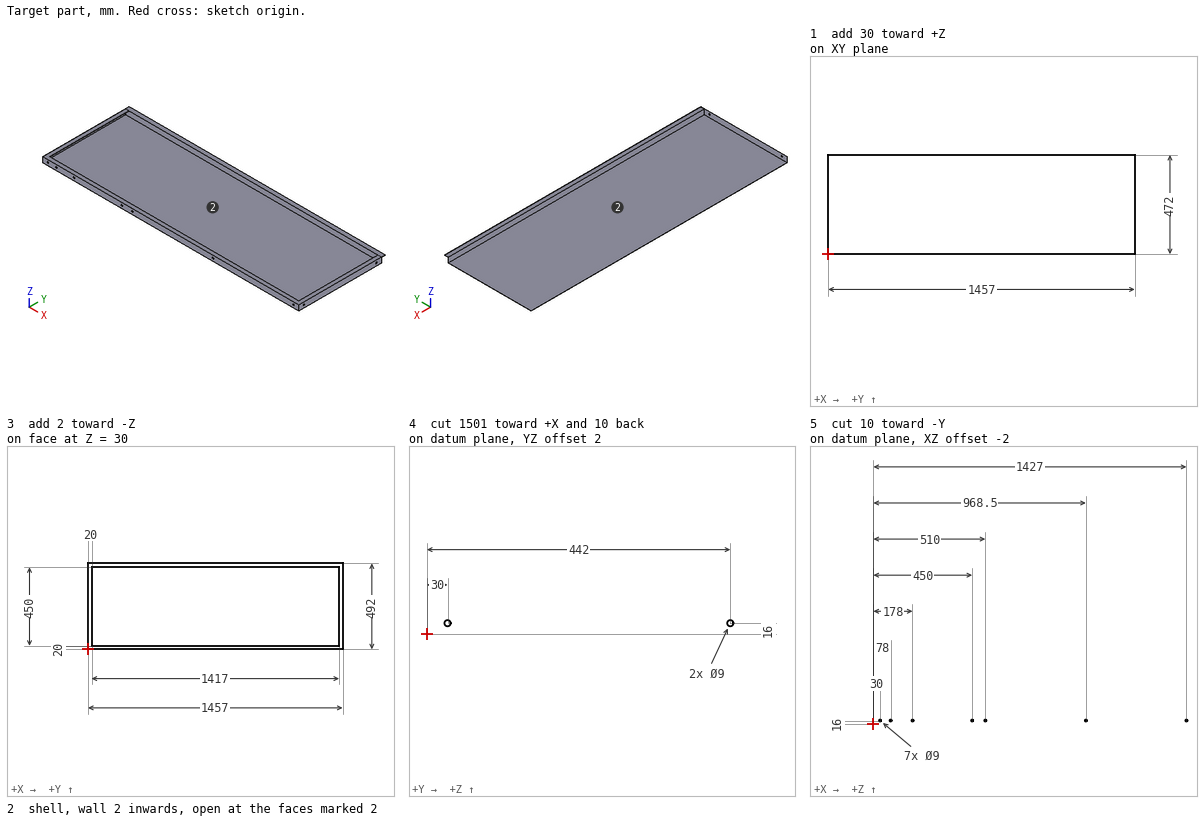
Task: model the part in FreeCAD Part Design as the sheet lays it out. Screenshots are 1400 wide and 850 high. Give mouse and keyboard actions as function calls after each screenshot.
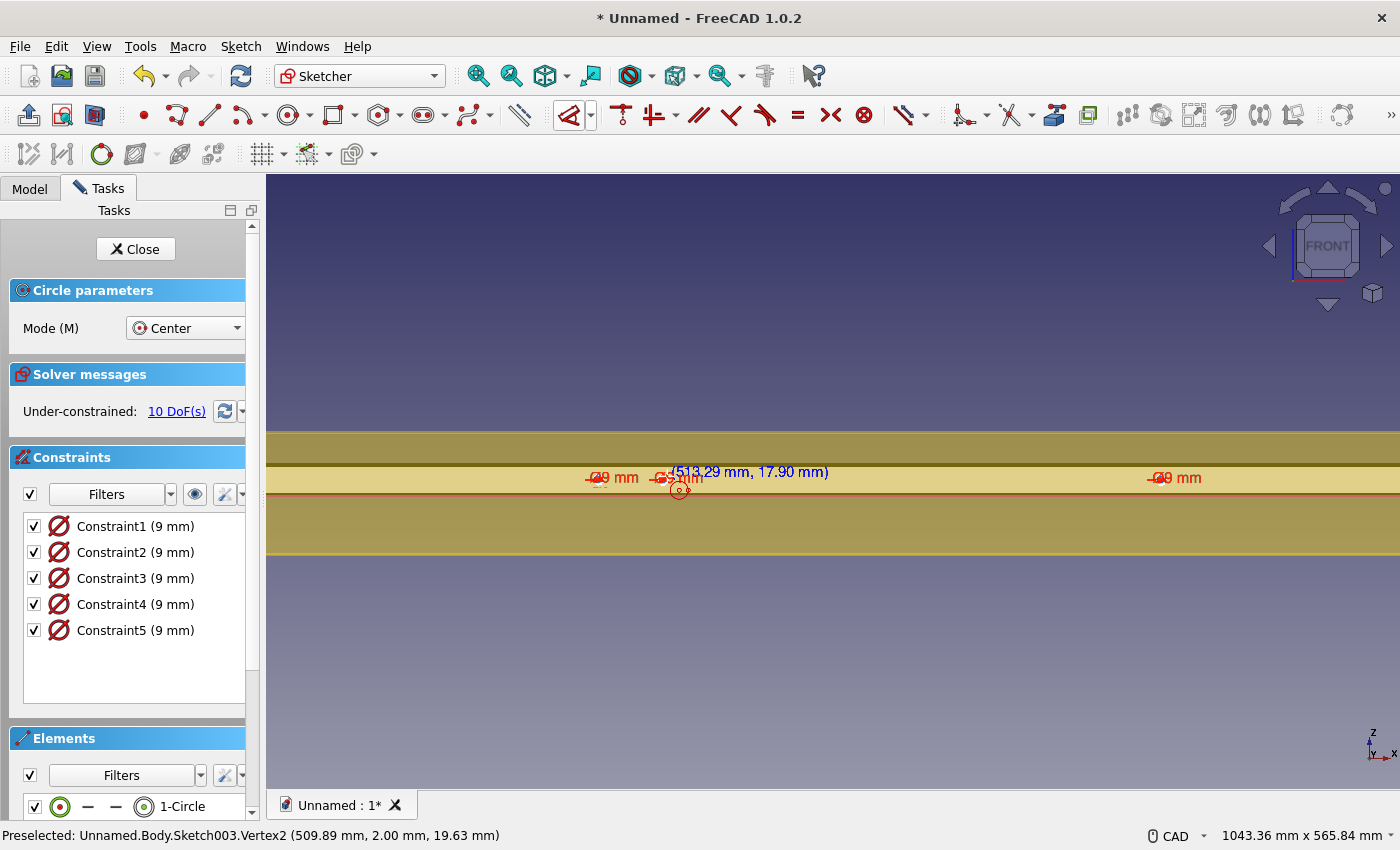
scroll(665, 478, down, 4)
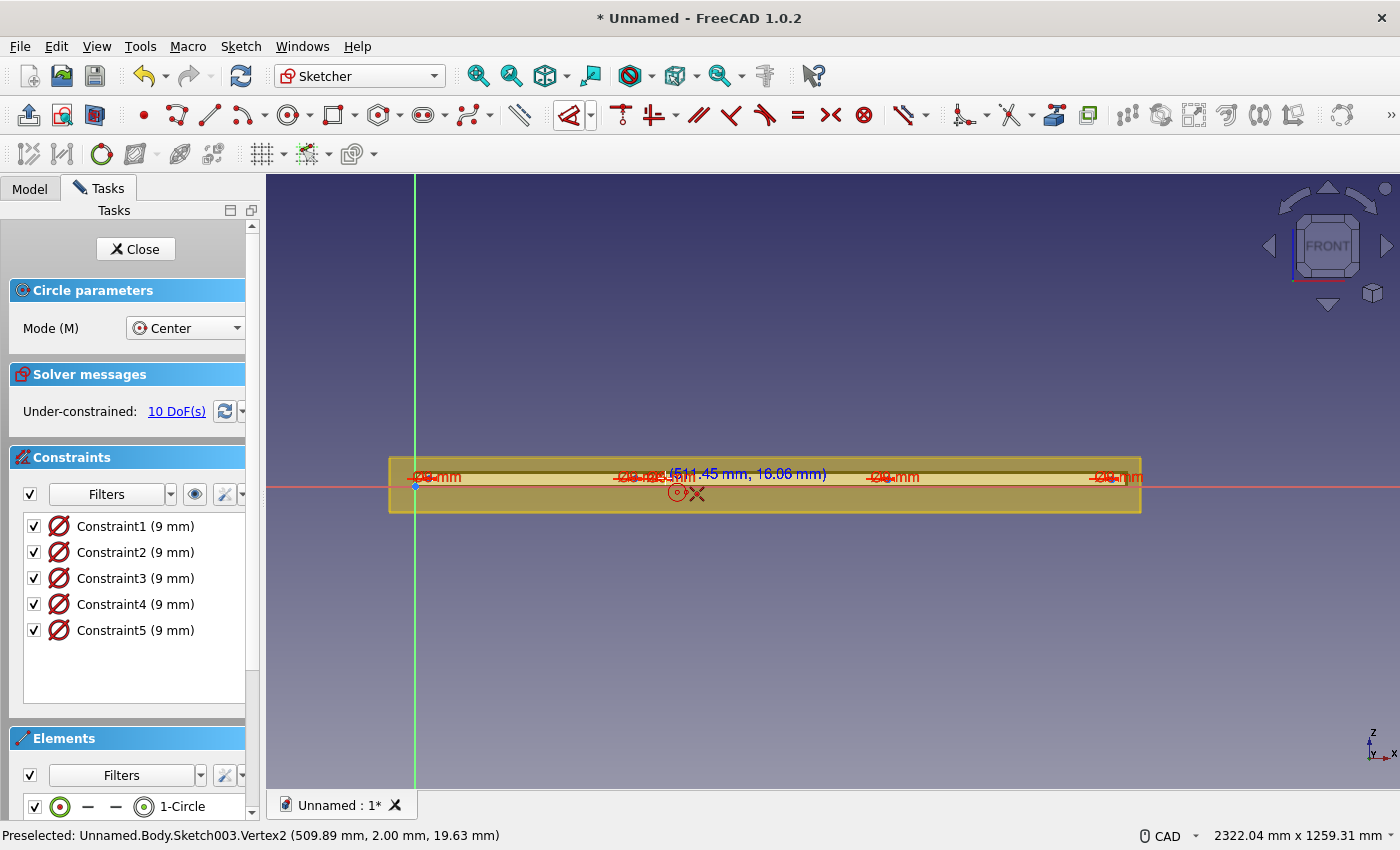
scroll(454, 479, up, 12)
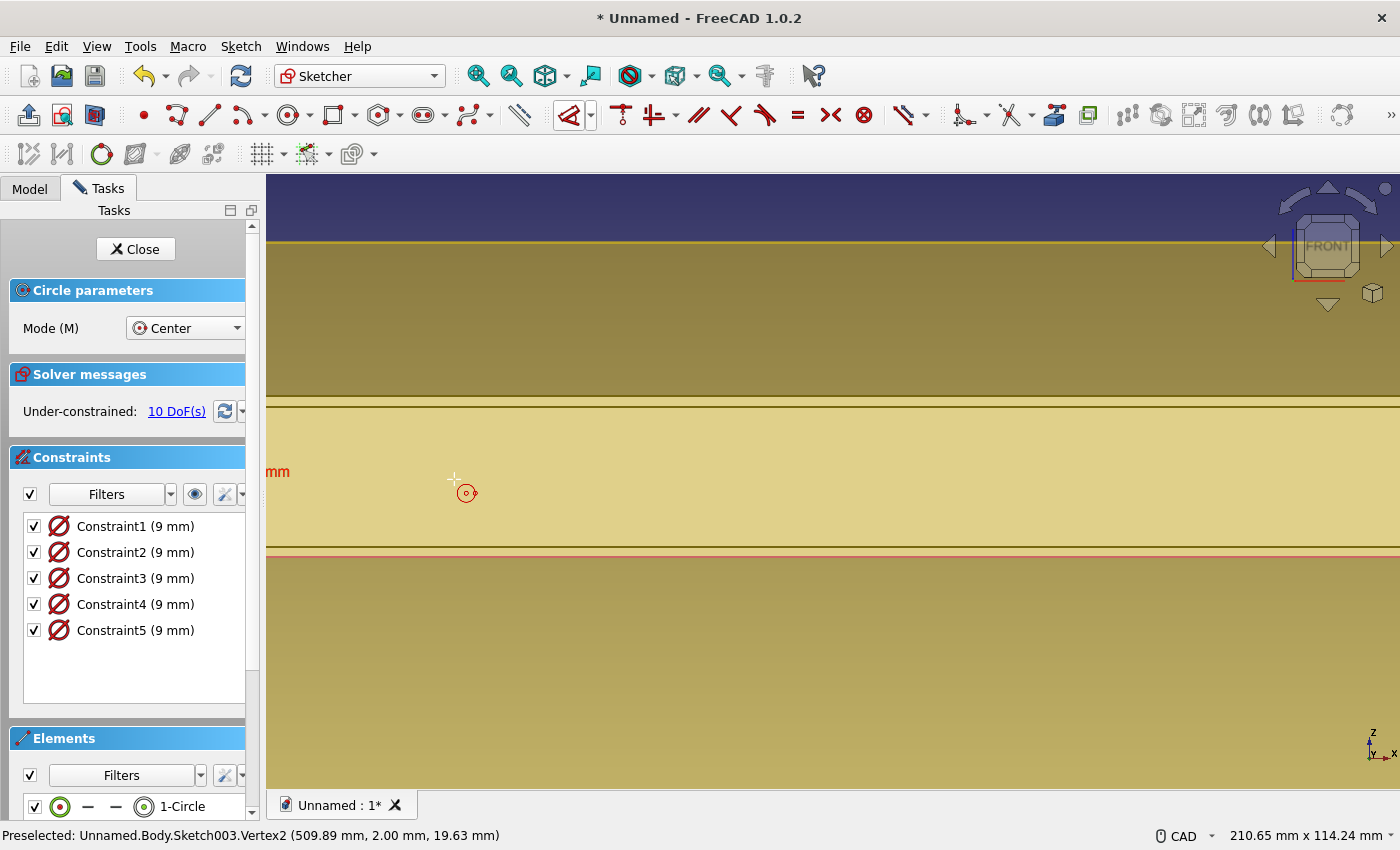
scroll(454, 479, down, 12)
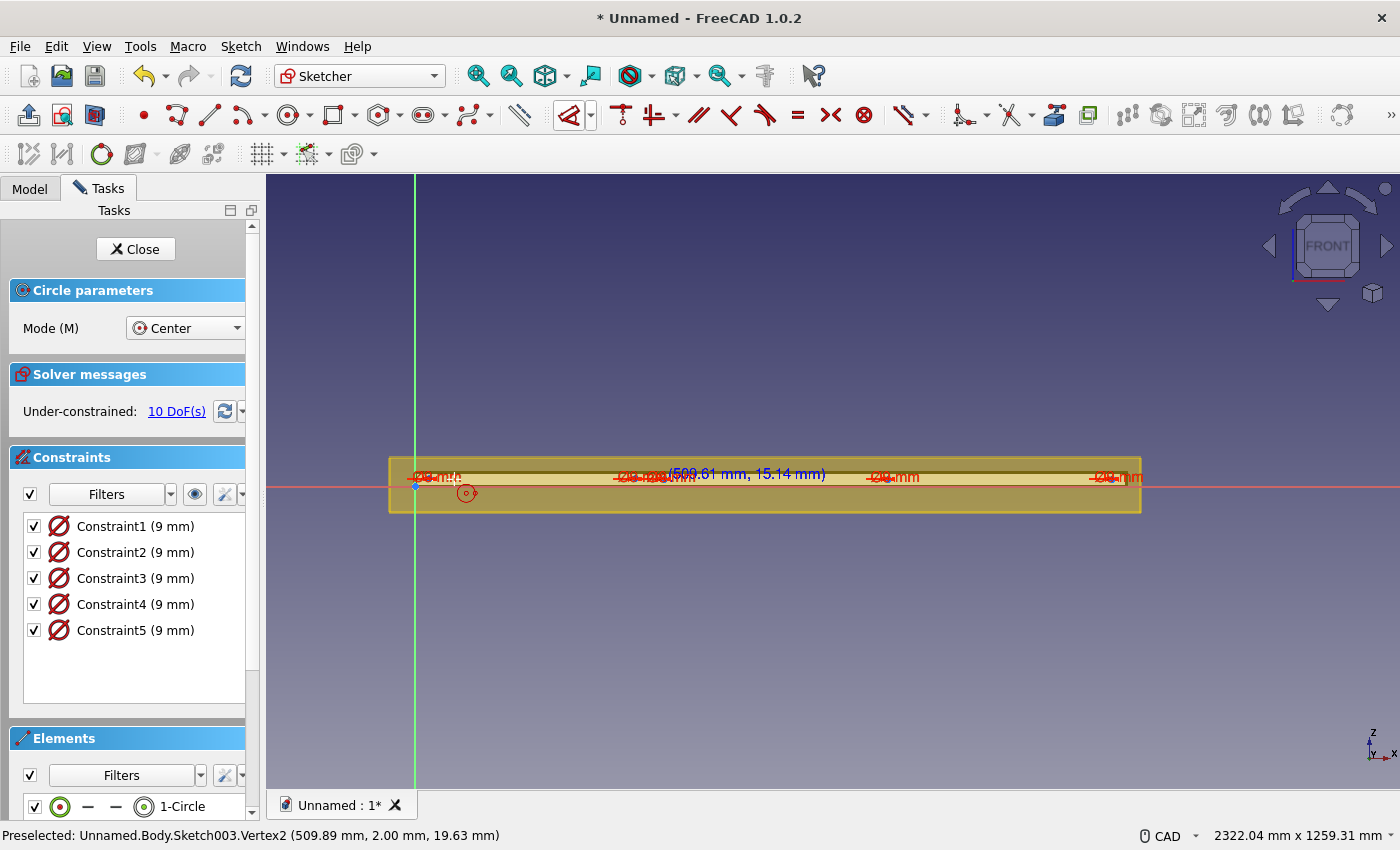
scroll(454, 479, up, 4)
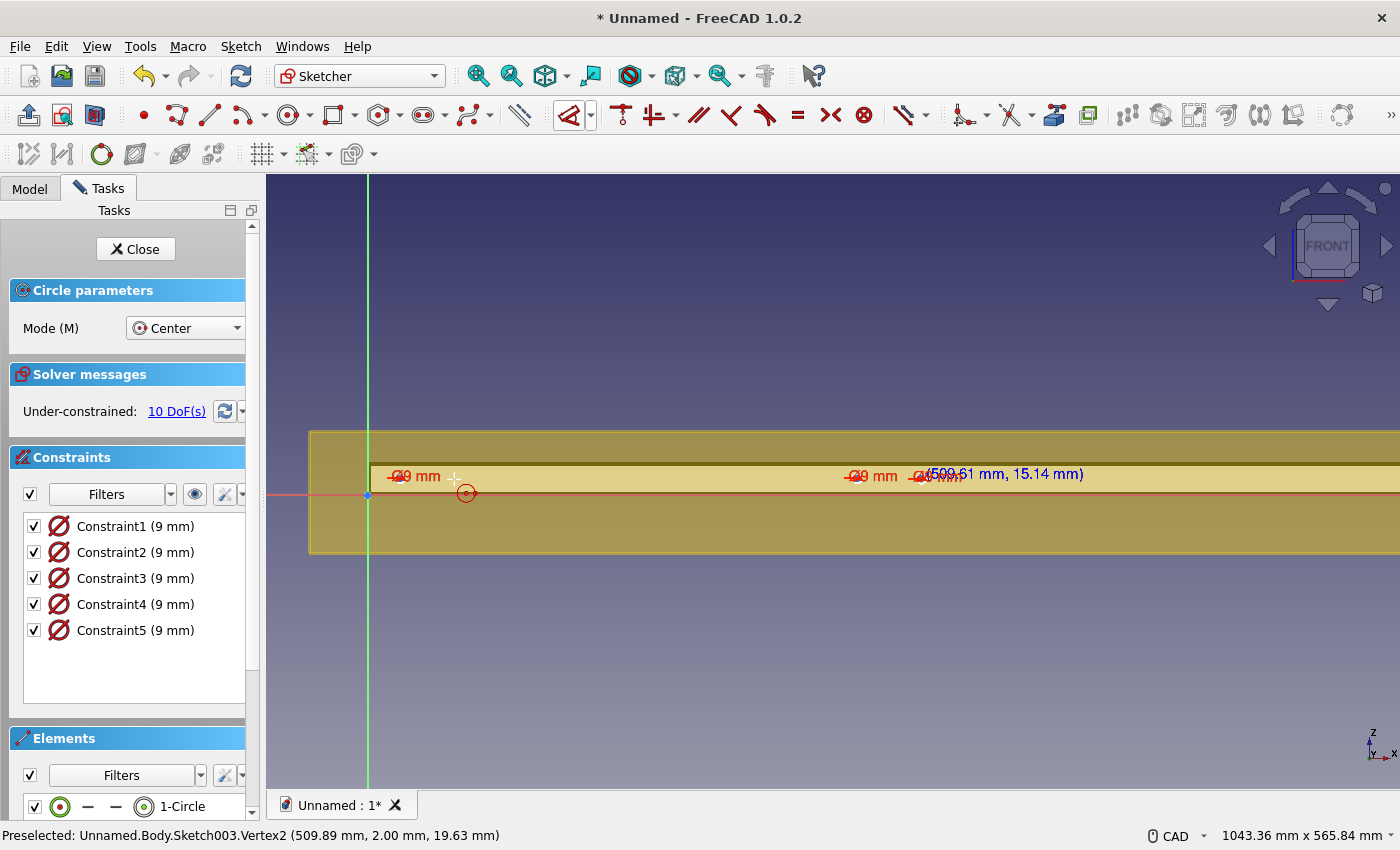
click(453, 478)
move(456, 474)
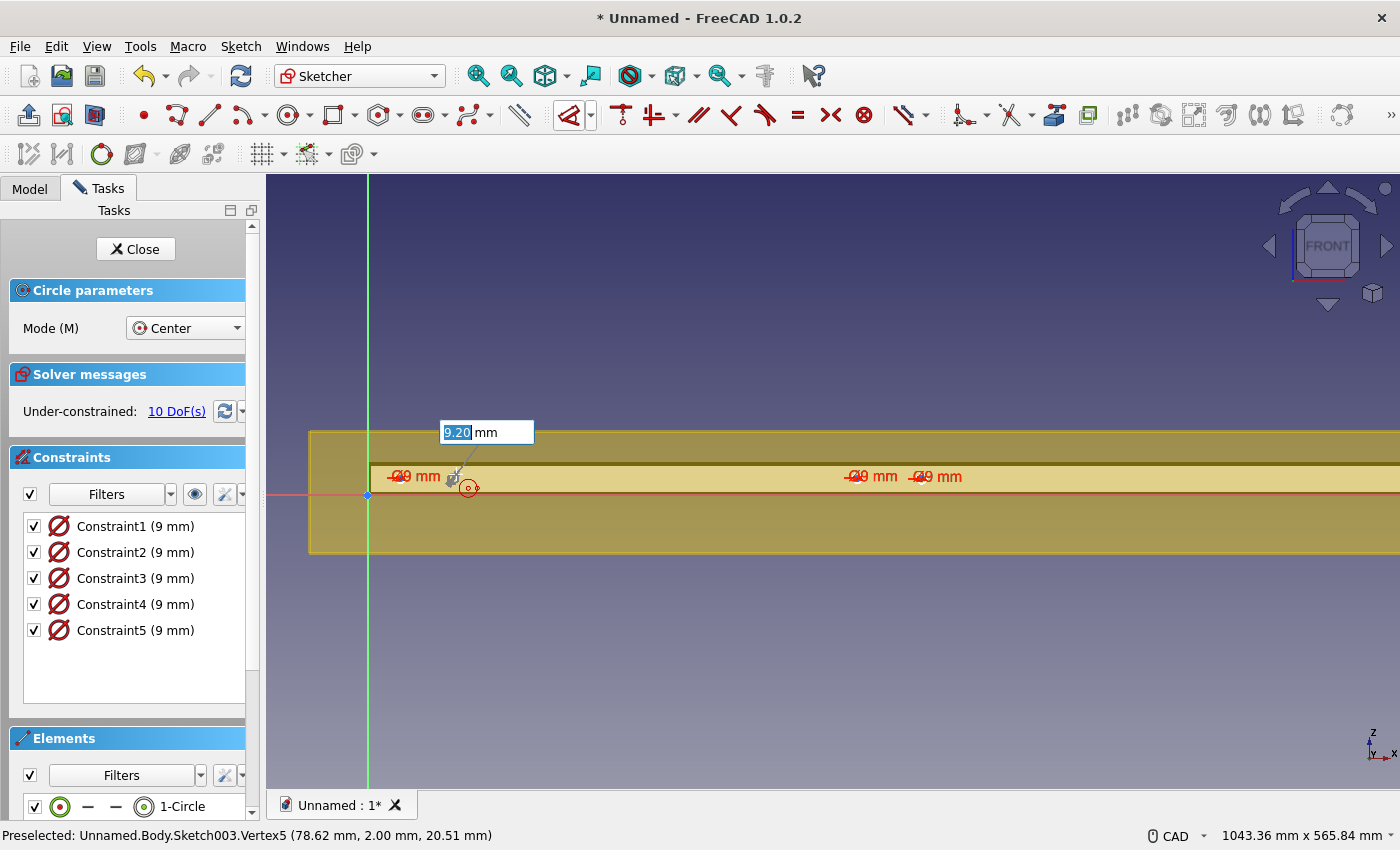
text(9)
key(Return)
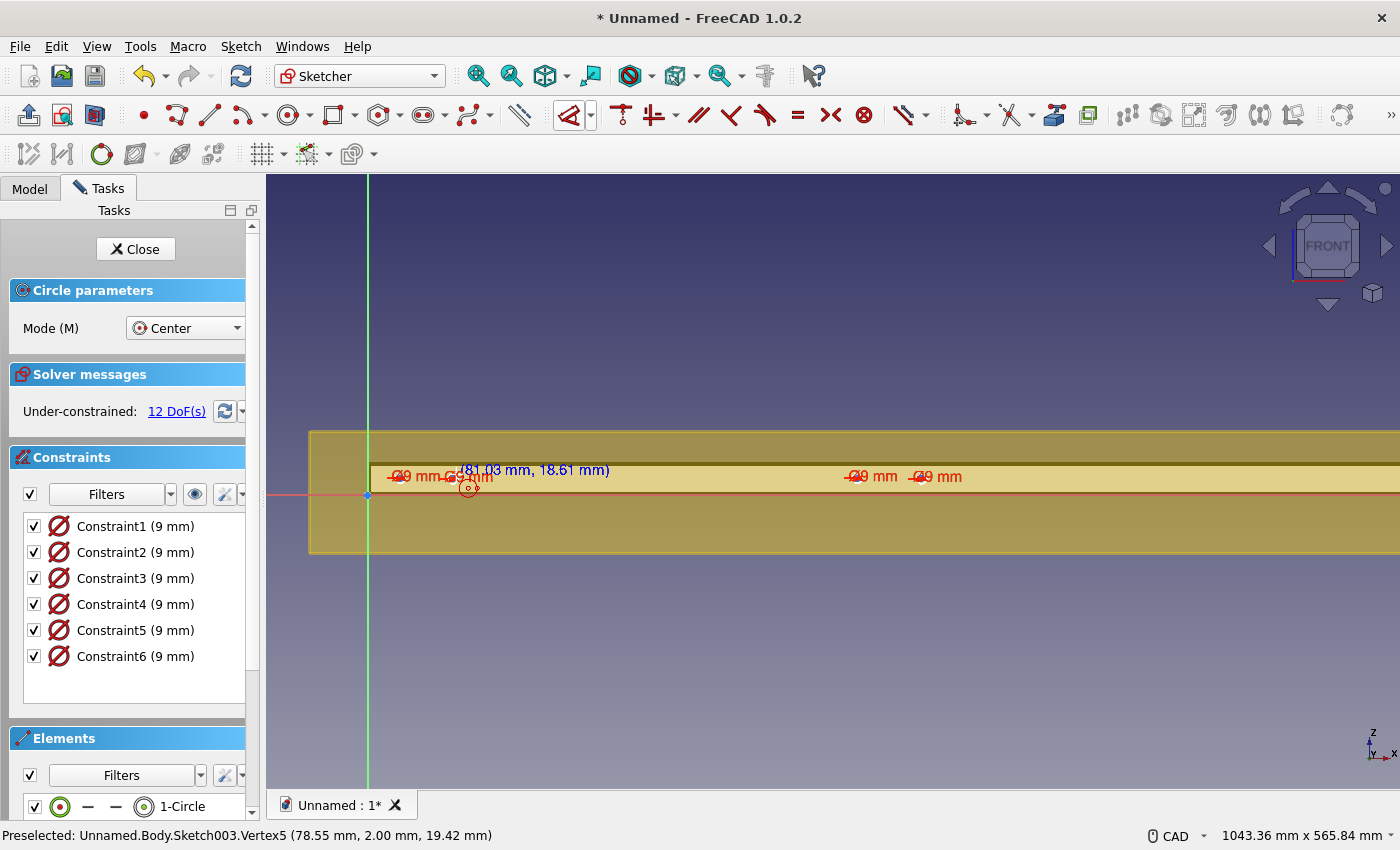
scroll(561, 478, up, 8)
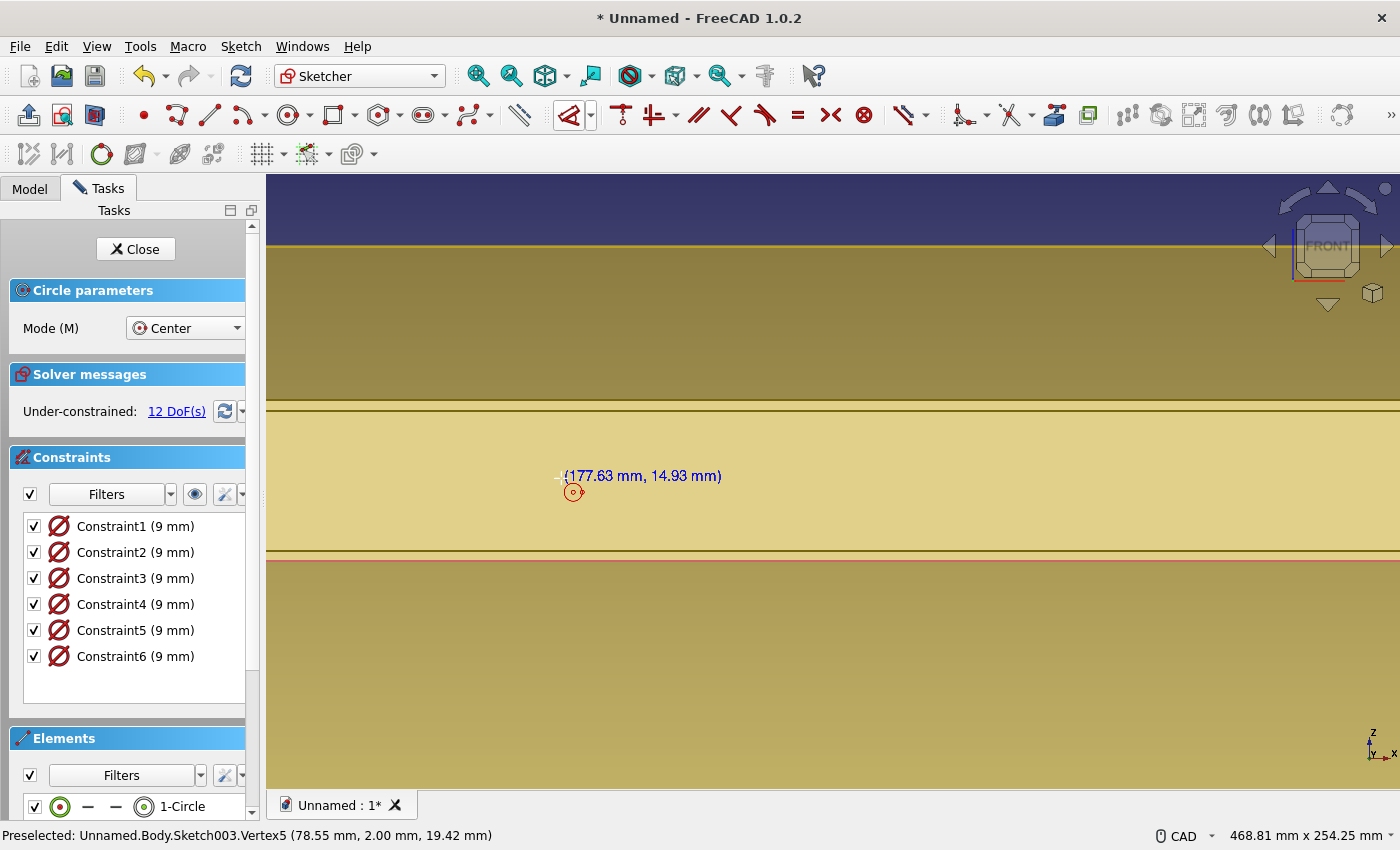
scroll(496, 479, down, 12)